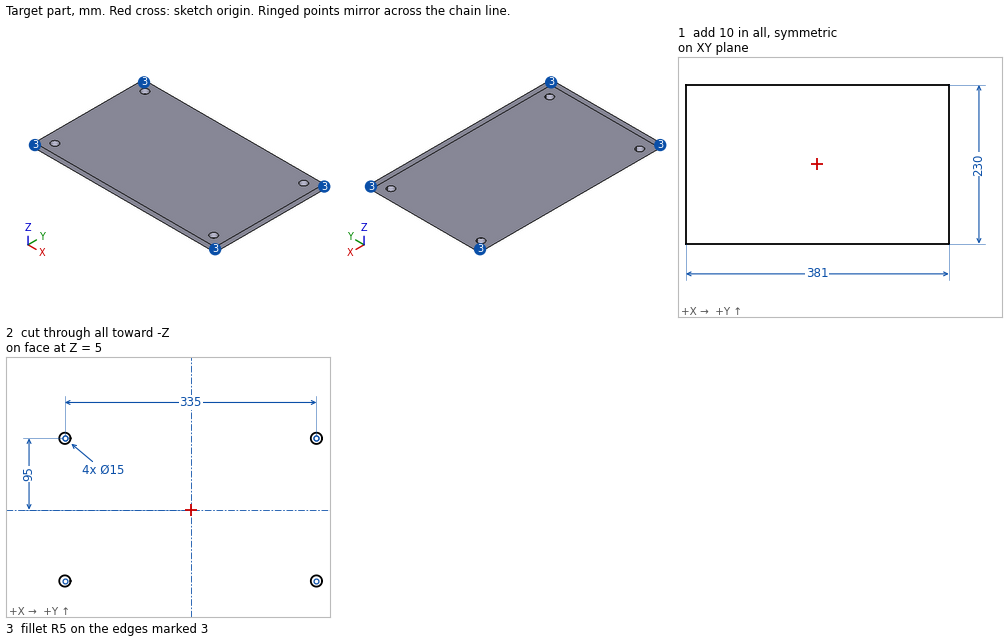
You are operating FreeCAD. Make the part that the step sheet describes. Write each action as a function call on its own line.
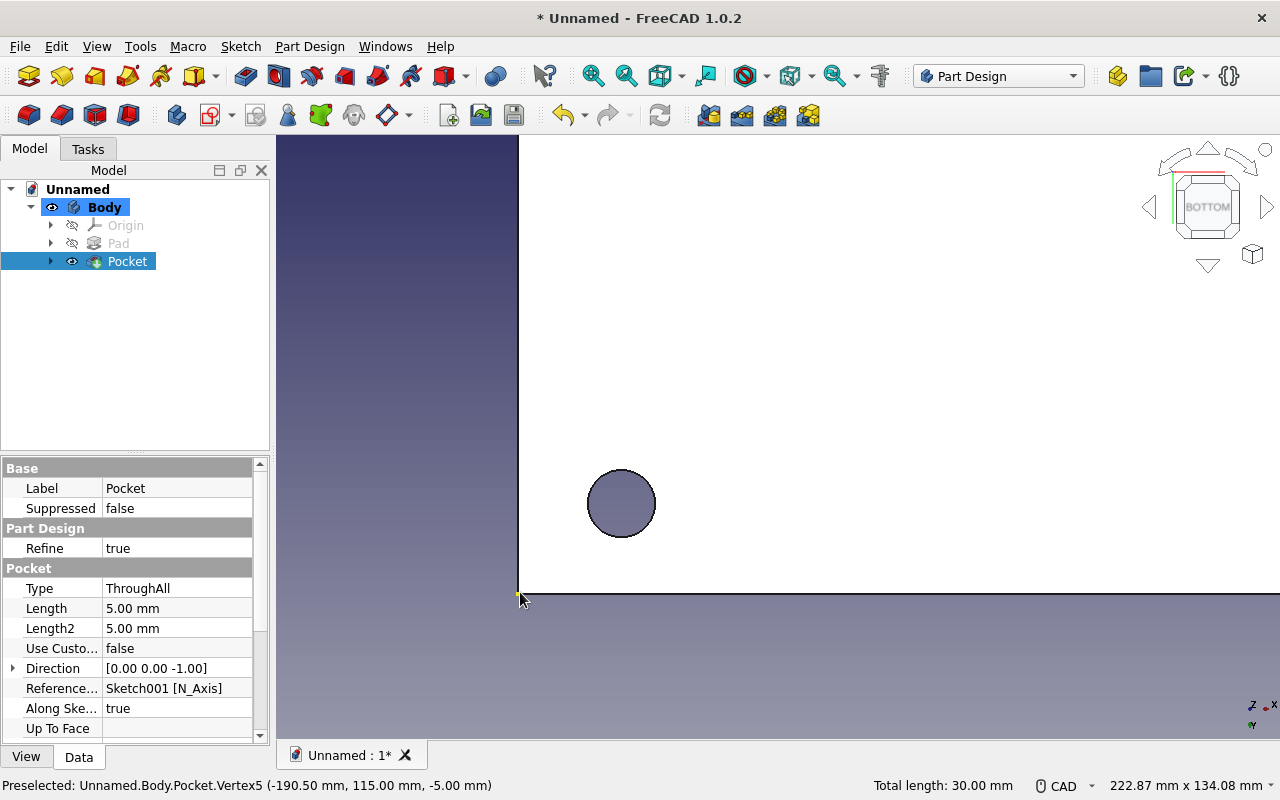
click(594, 76)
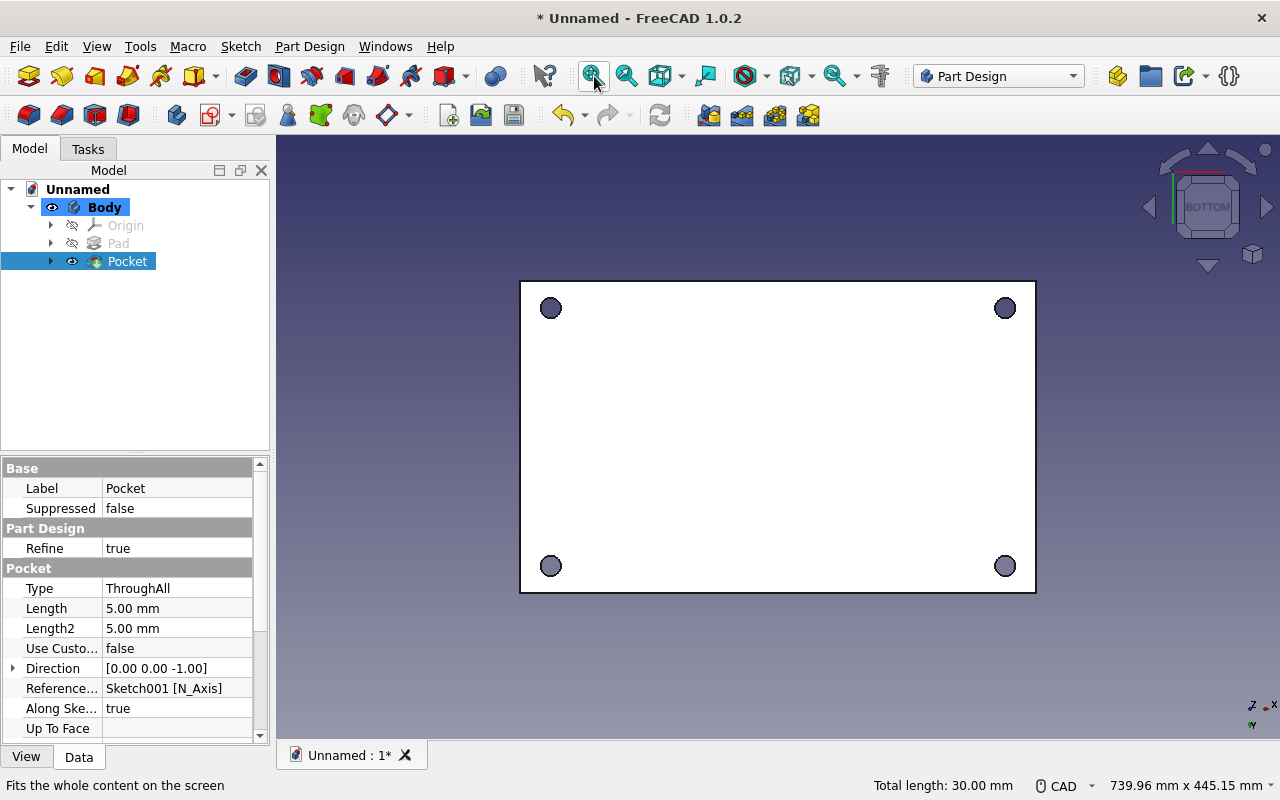
key(4)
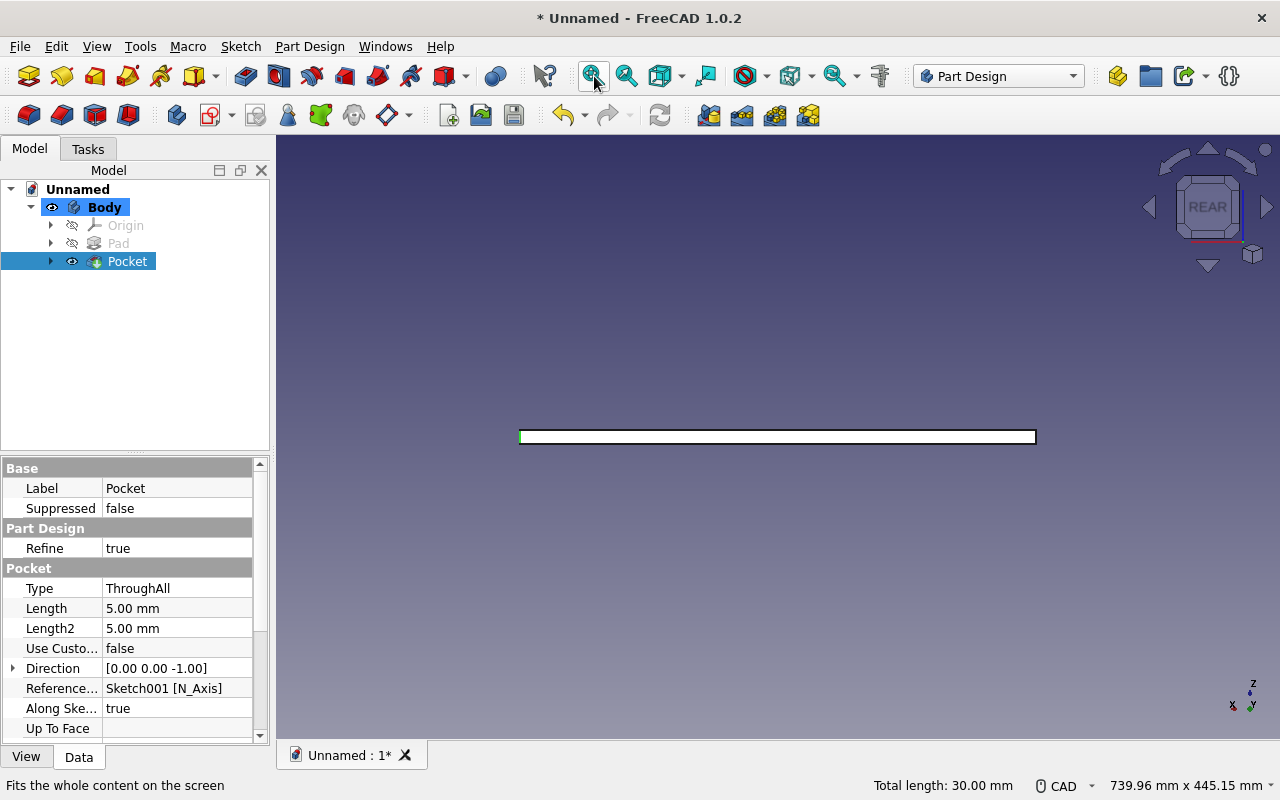
click(1036, 436, ctrl)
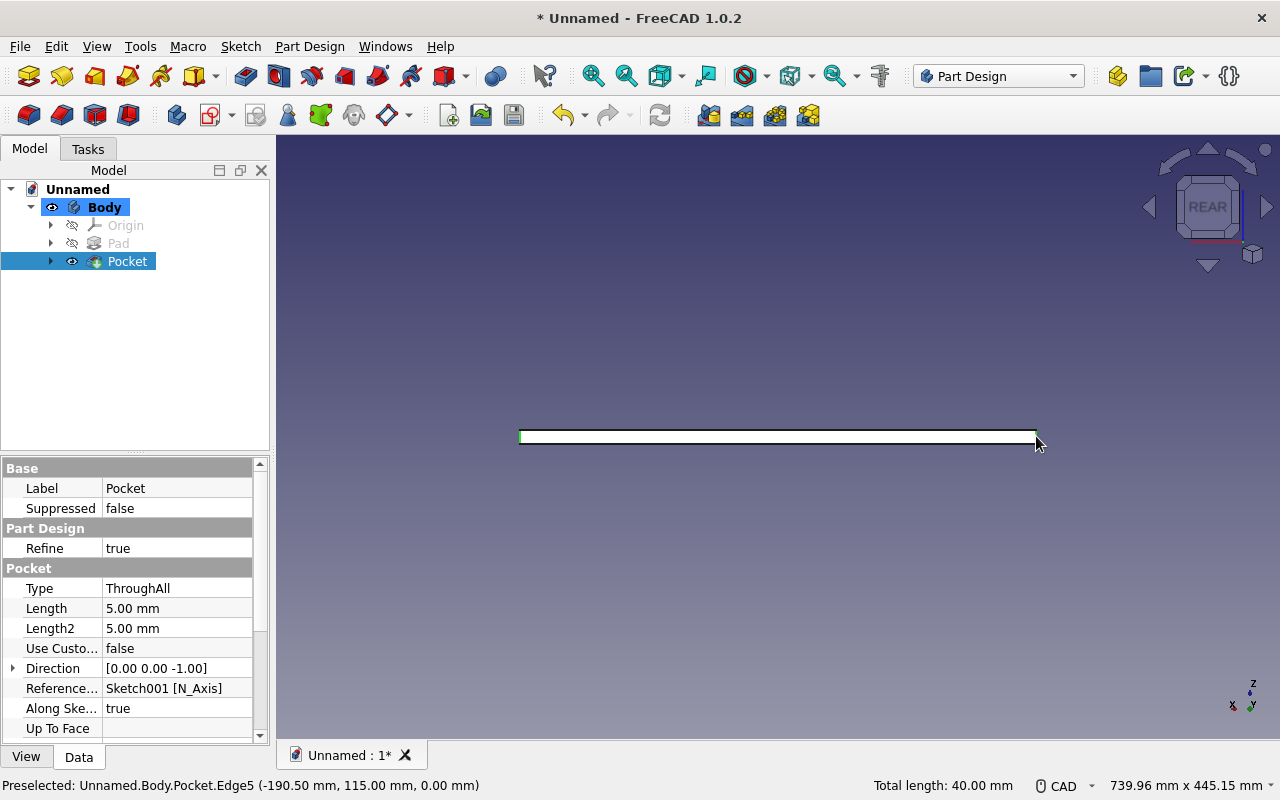
click(29, 116)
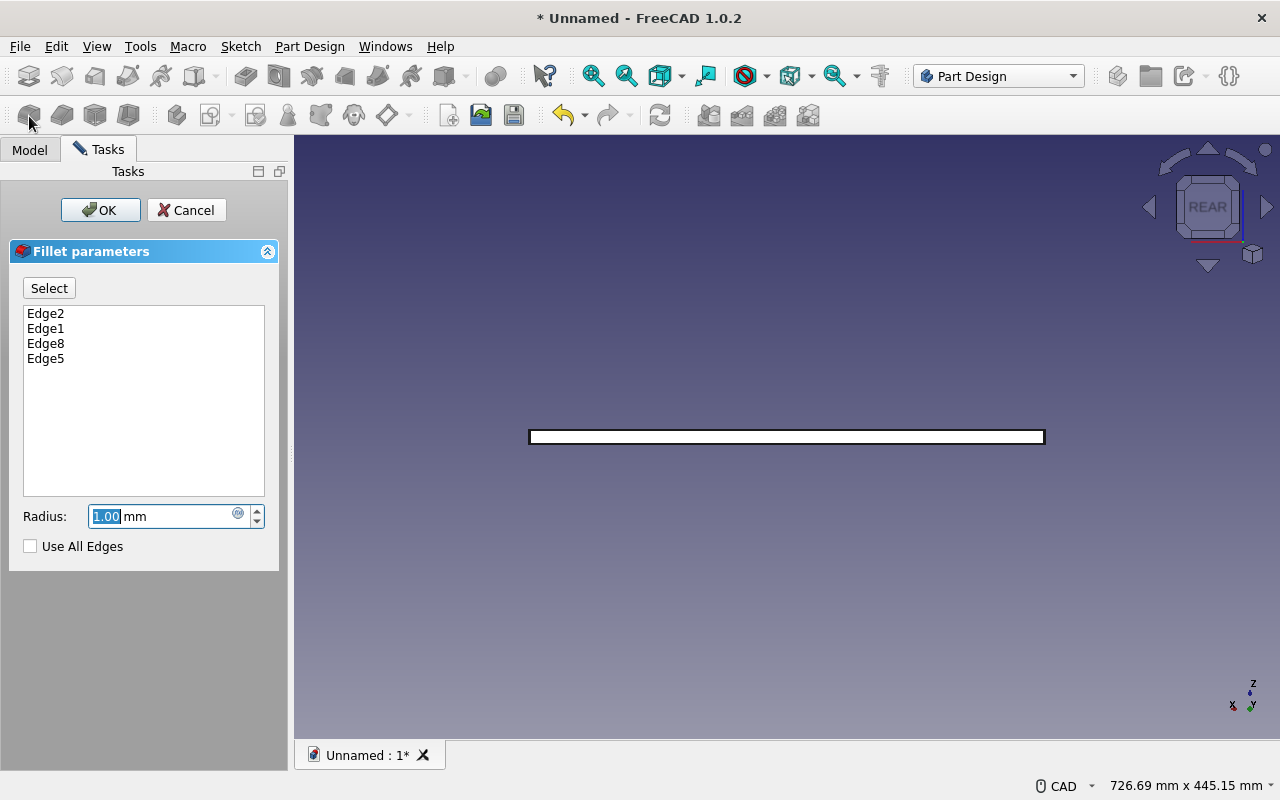
text(5)
key(Tab)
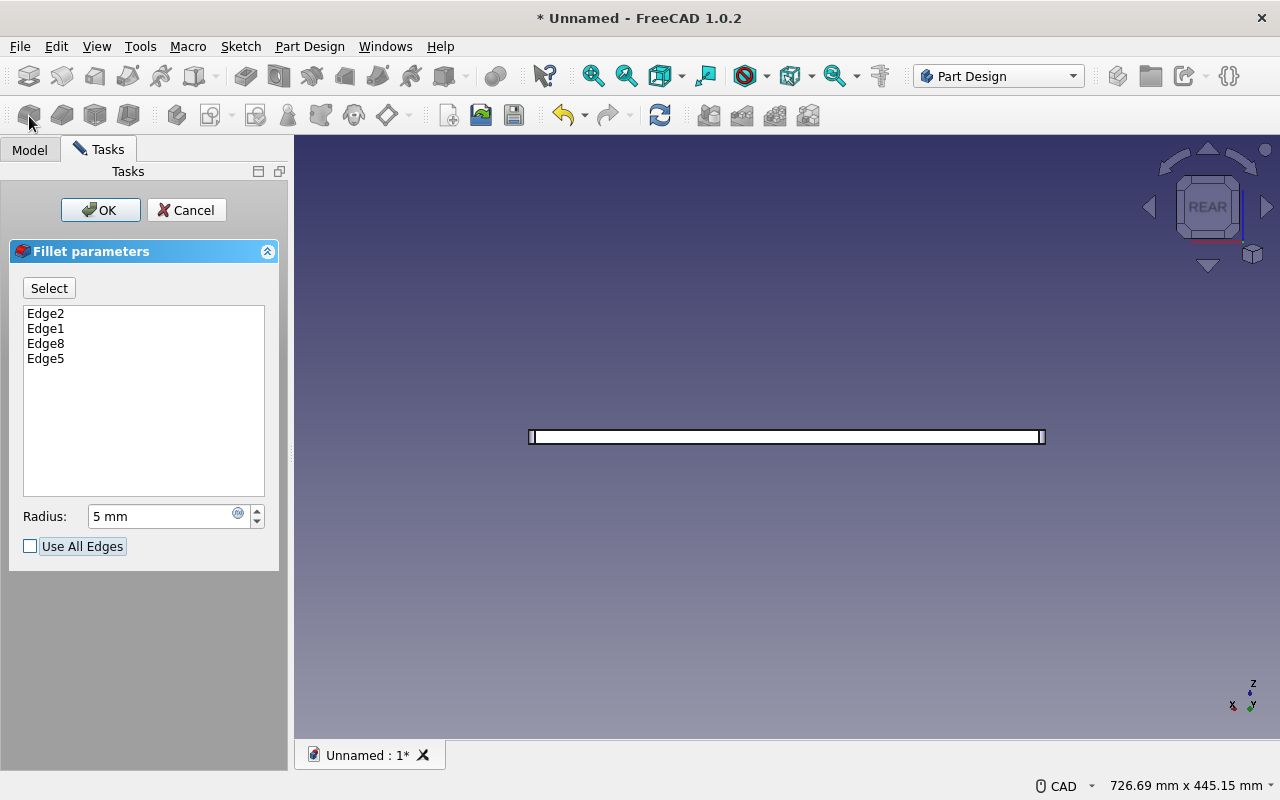
click(101, 210)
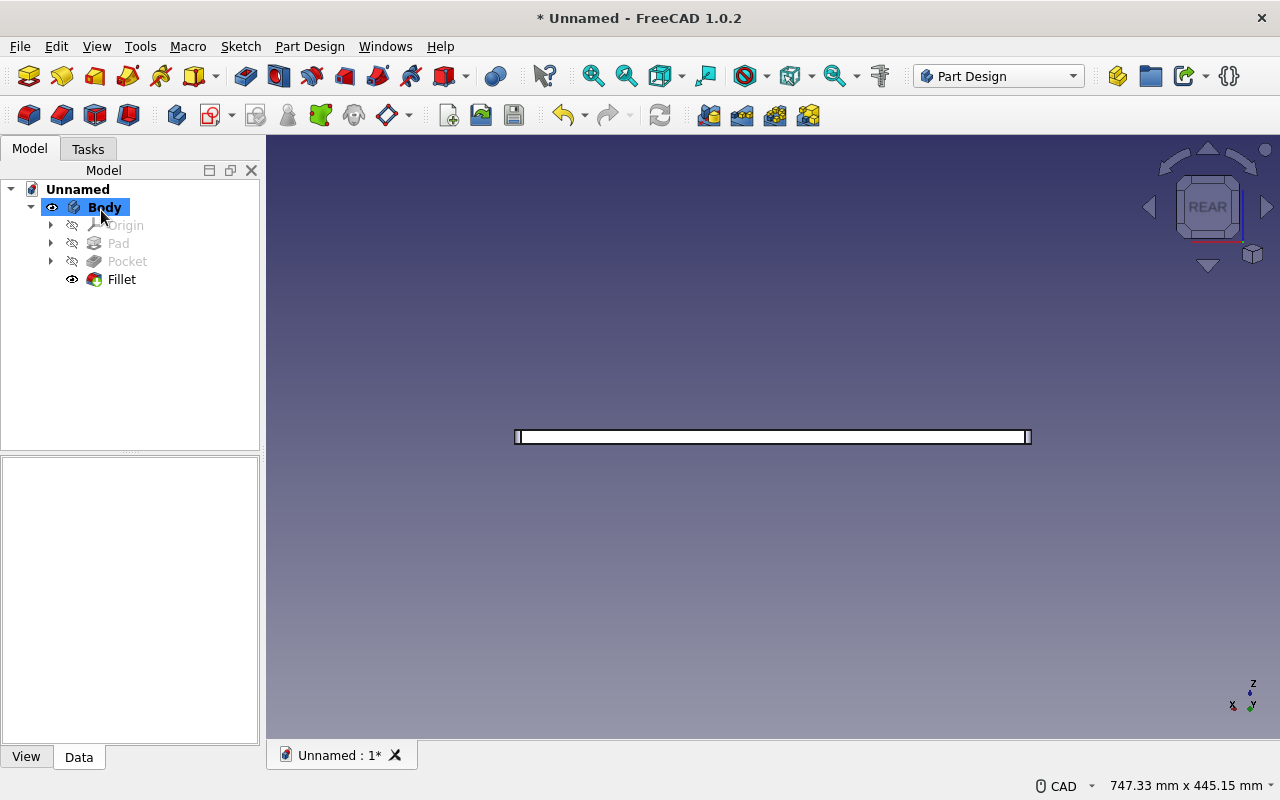
key(0)